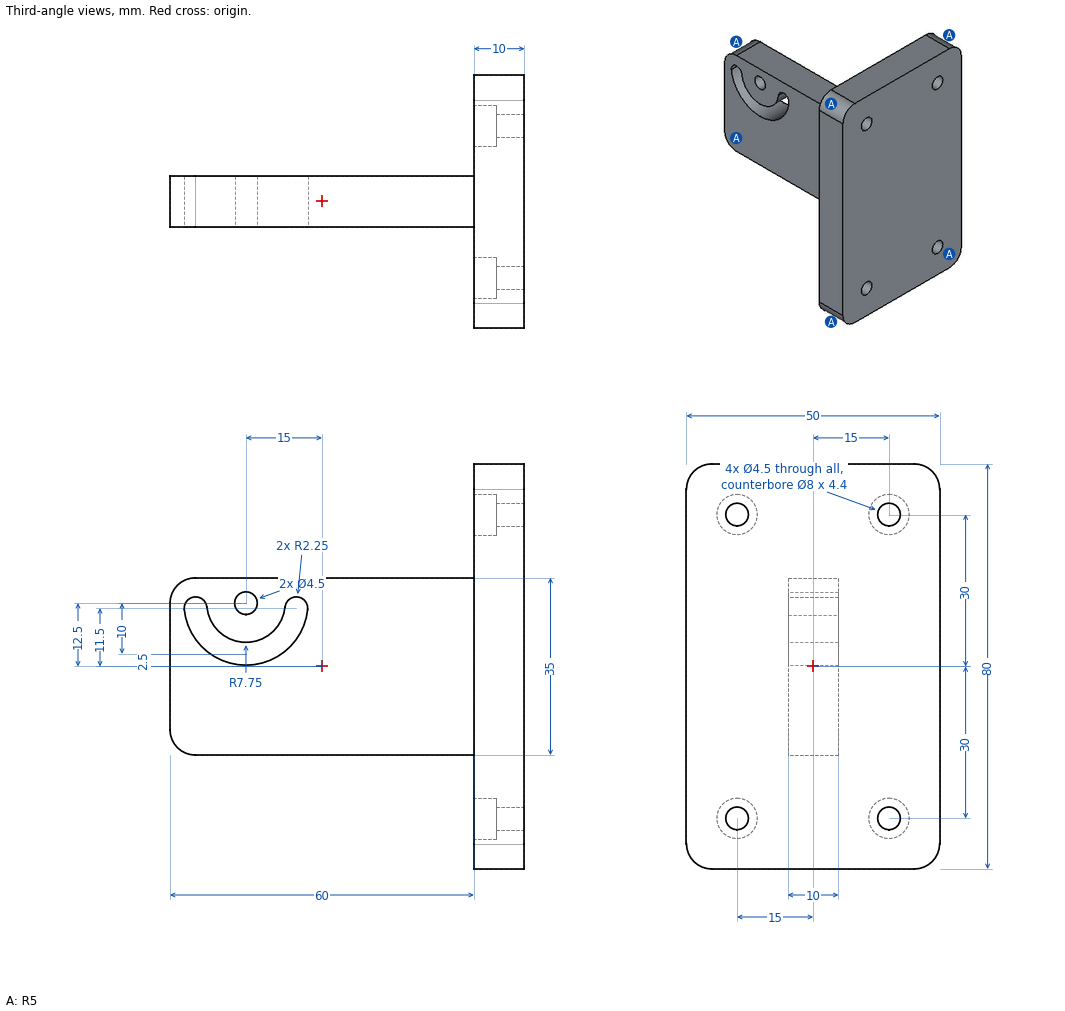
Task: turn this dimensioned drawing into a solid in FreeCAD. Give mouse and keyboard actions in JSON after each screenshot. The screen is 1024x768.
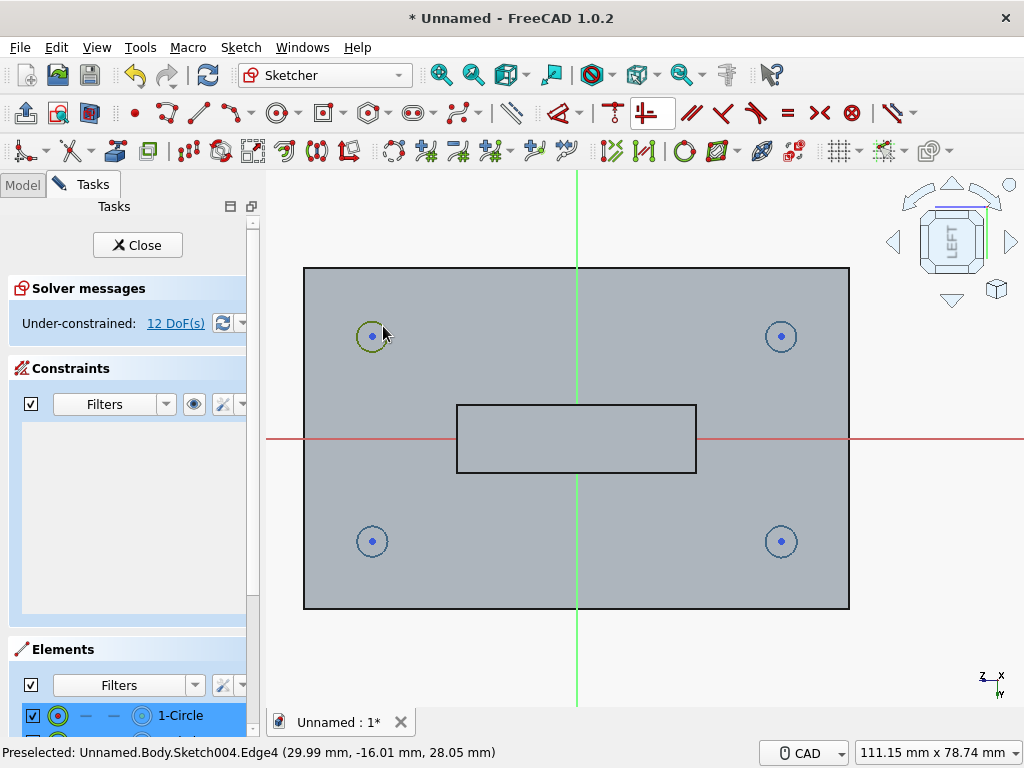
{"action": "left_click", "coordinate": [788, 114]}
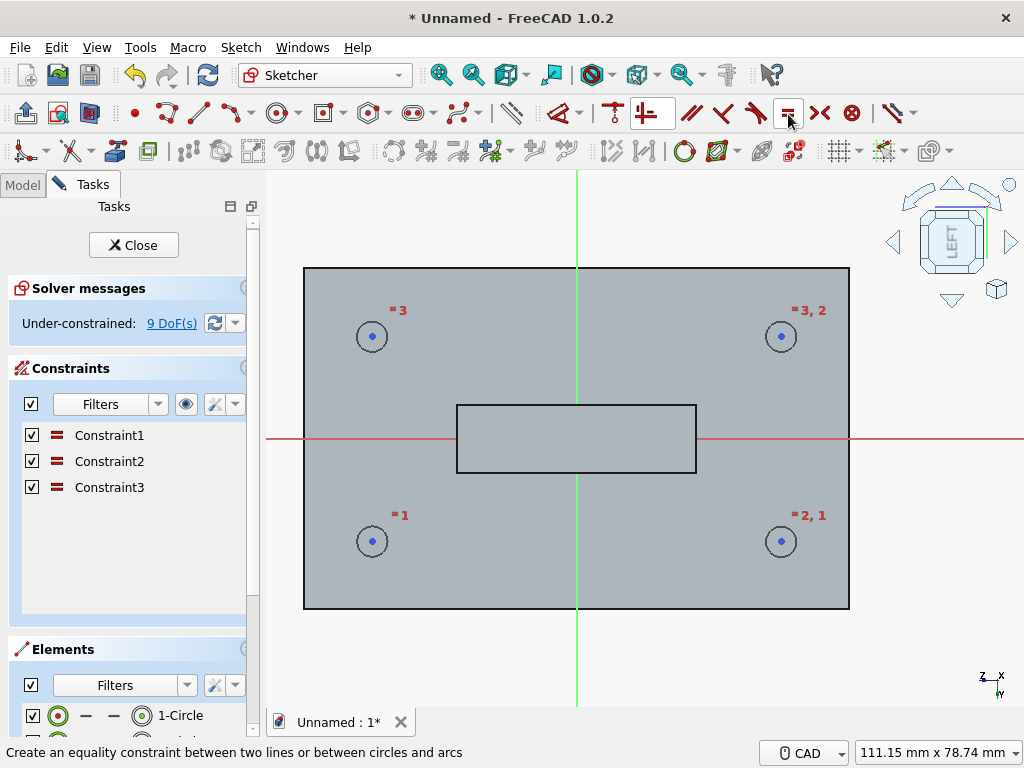
{"action": "left_click", "coordinate": [372, 542]}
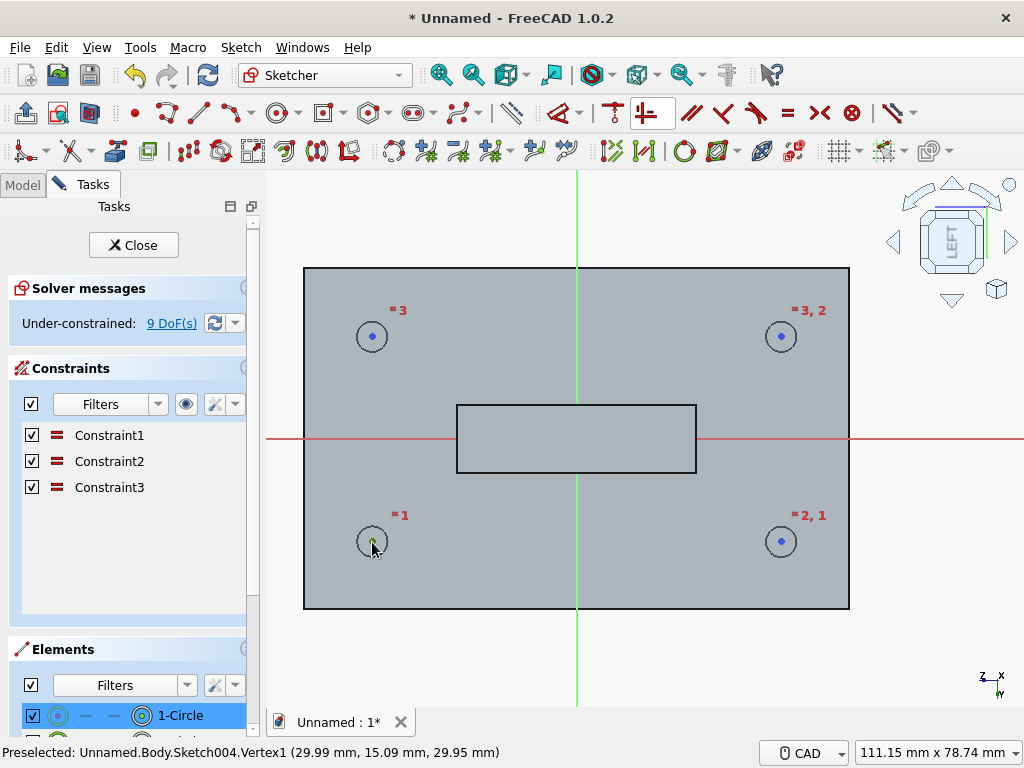
{"action": "left_click", "coordinate": [781, 542]}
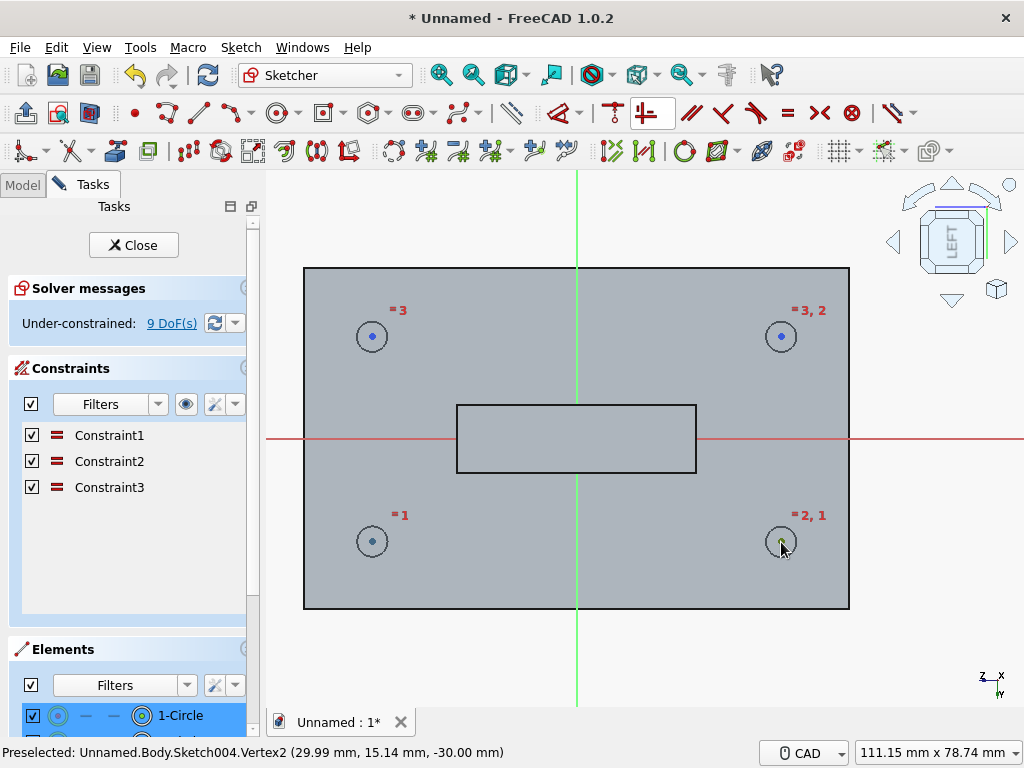
{"action": "left_click", "coordinate": [670, 114]}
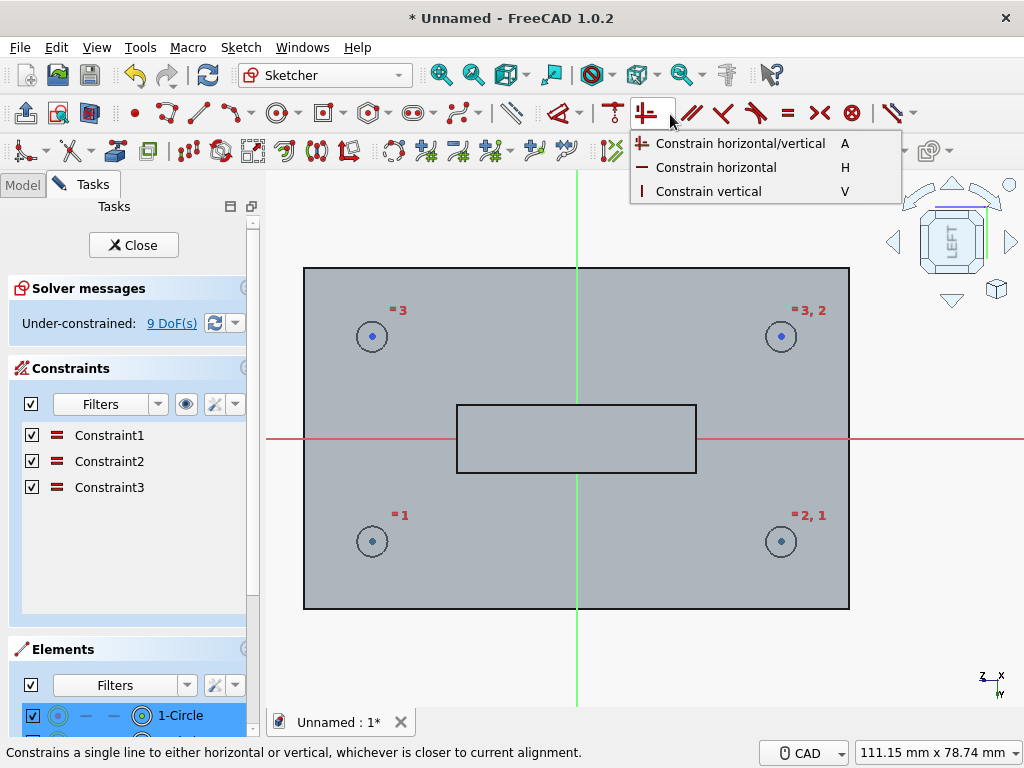
{"action": "left_click", "coordinate": [766, 167]}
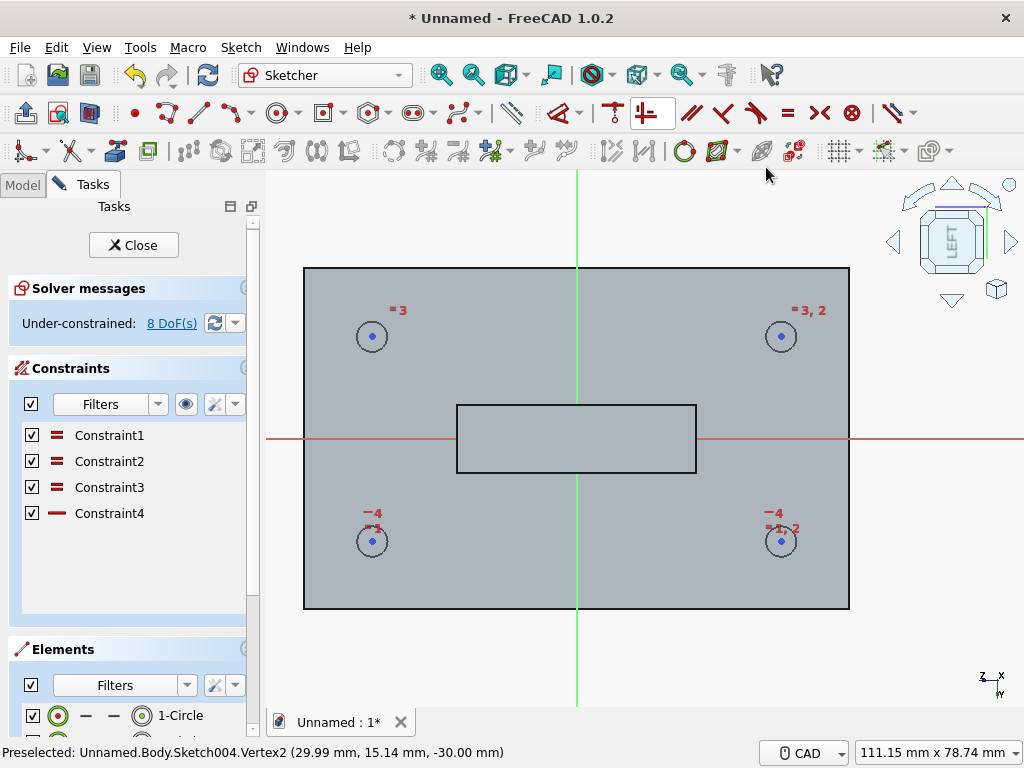
{"action": "left_click", "coordinate": [781, 542]}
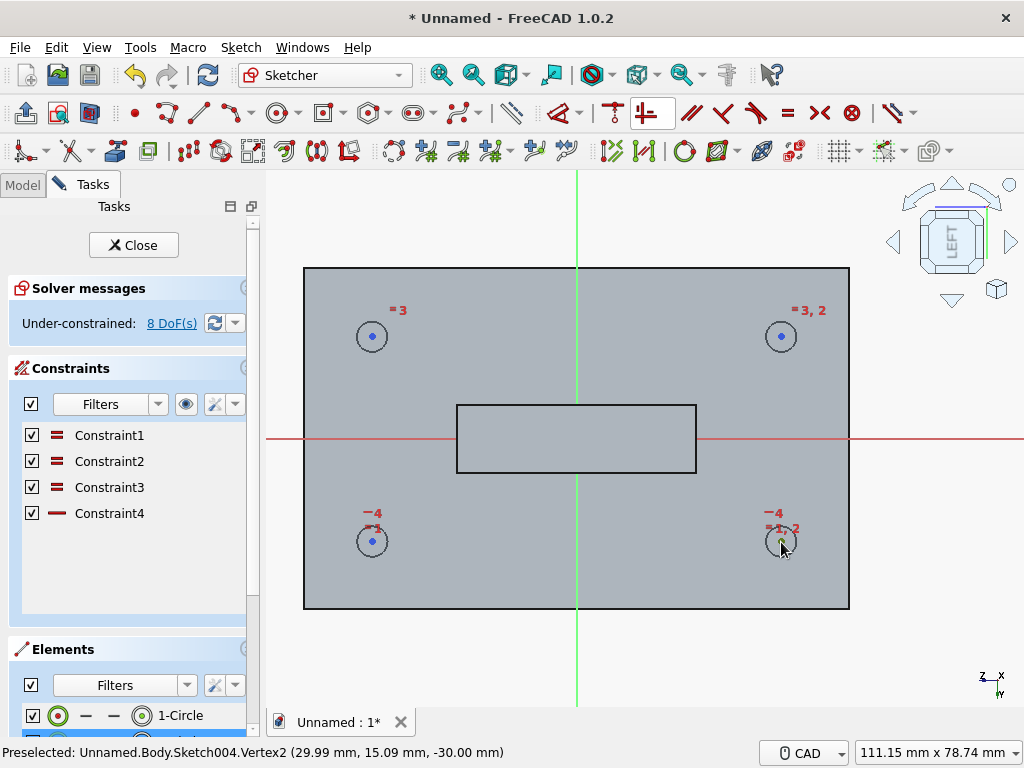
{"action": "left_click", "coordinate": [781, 337]}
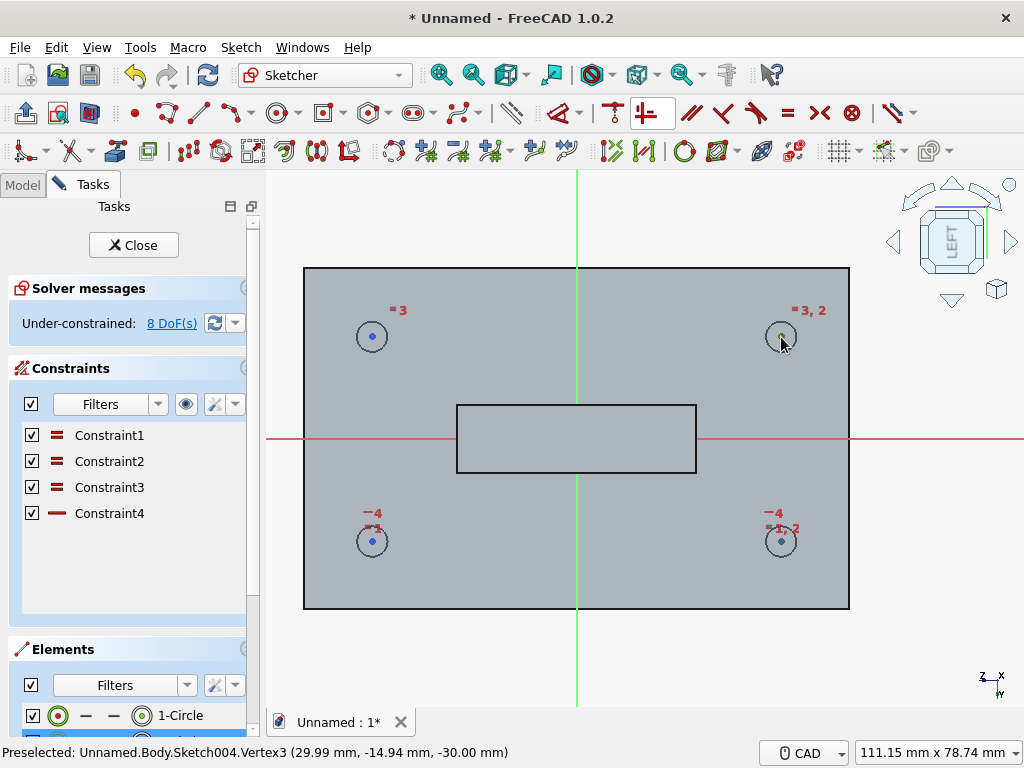
{"action": "left_click", "coordinate": [670, 114]}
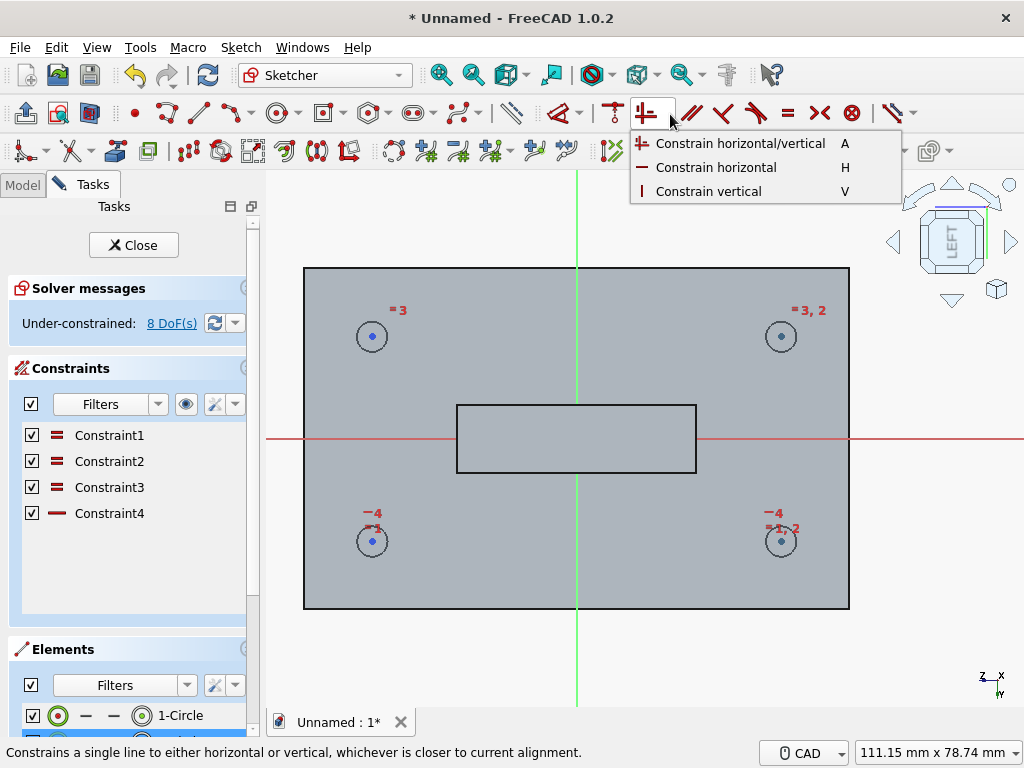
{"action": "left_click", "coordinate": [766, 191]}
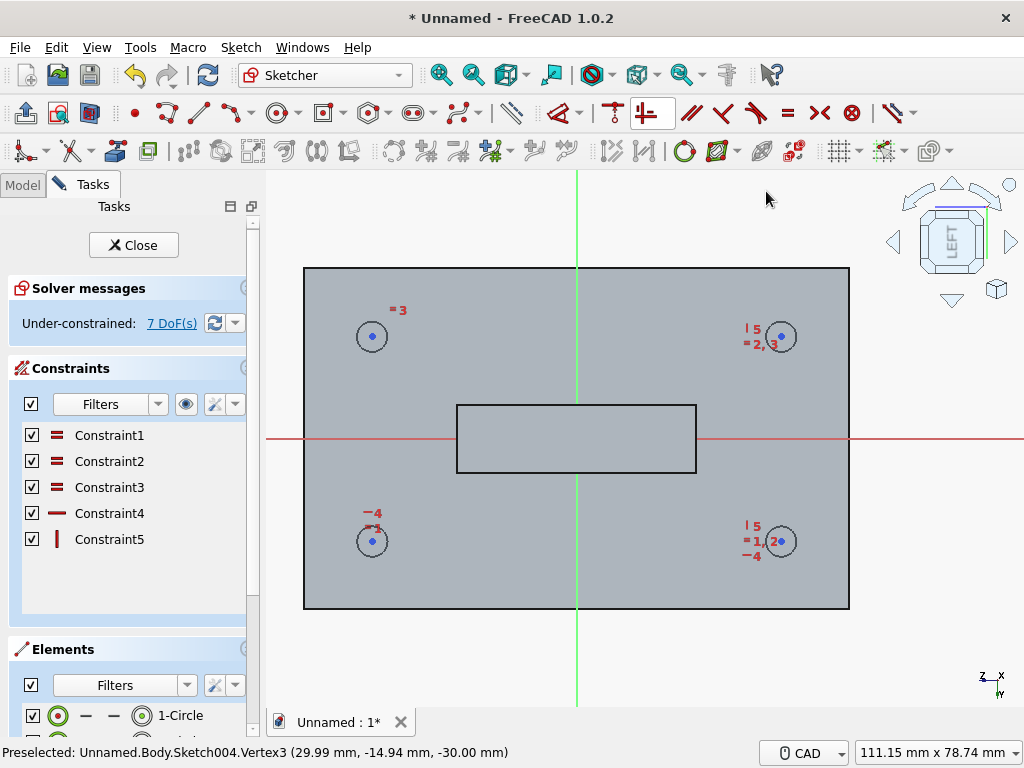
{"action": "left_click", "coordinate": [372, 542]}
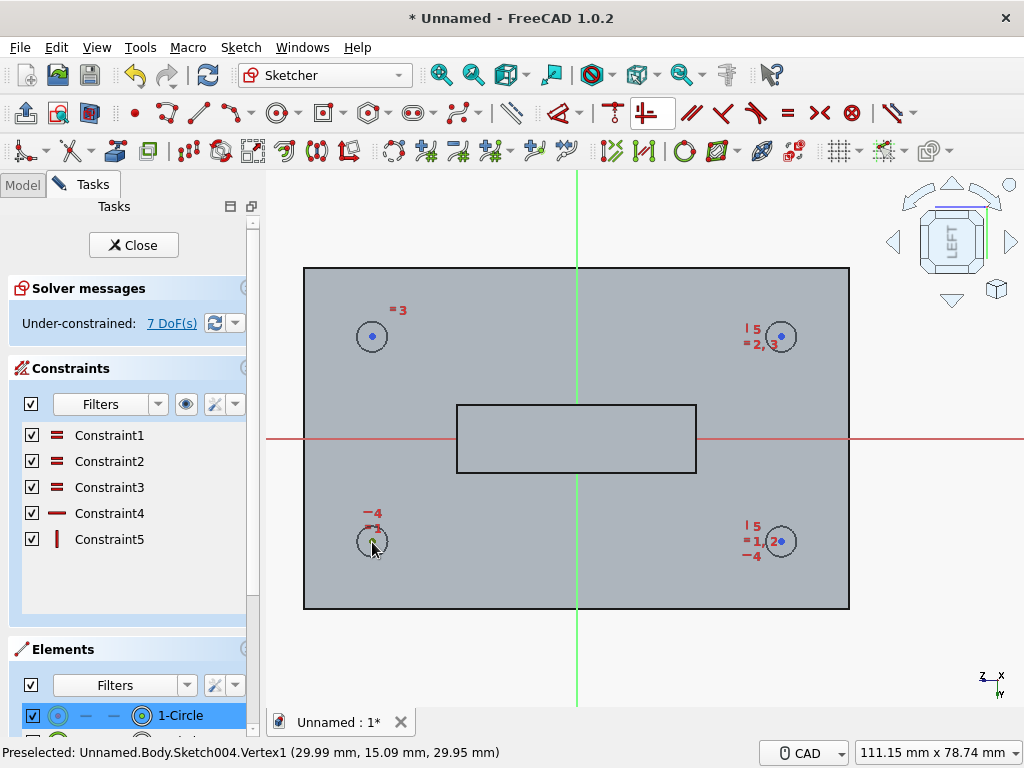
{"action": "left_click", "coordinate": [372, 337]}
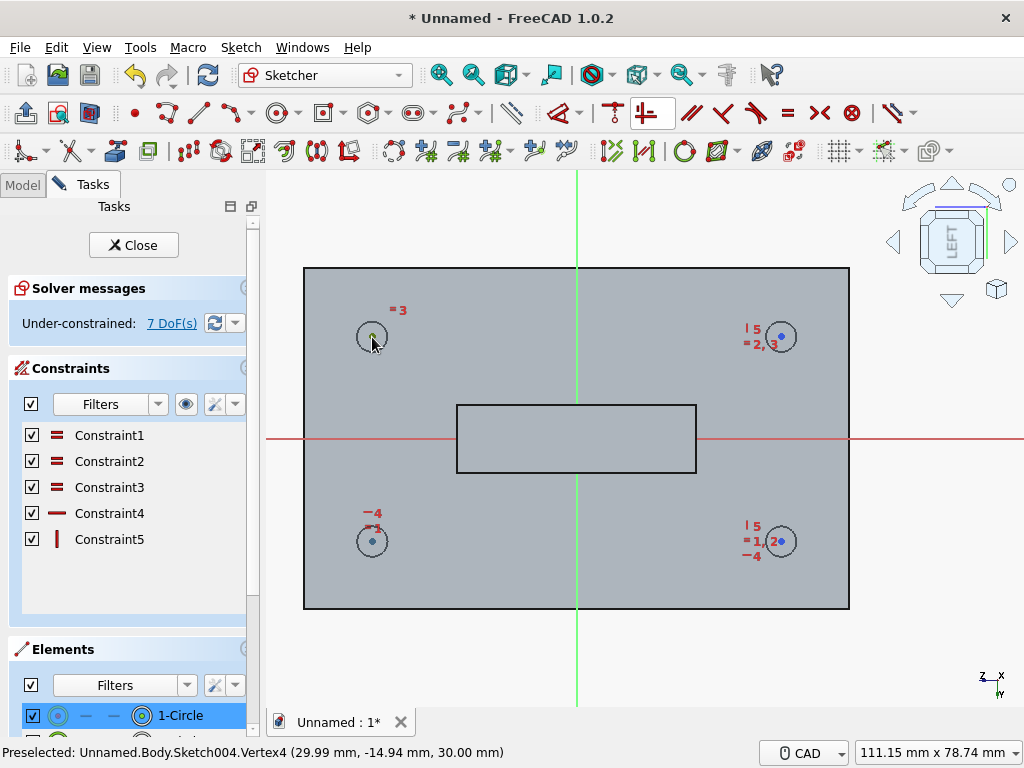
{"action": "left_click", "coordinate": [670, 114]}